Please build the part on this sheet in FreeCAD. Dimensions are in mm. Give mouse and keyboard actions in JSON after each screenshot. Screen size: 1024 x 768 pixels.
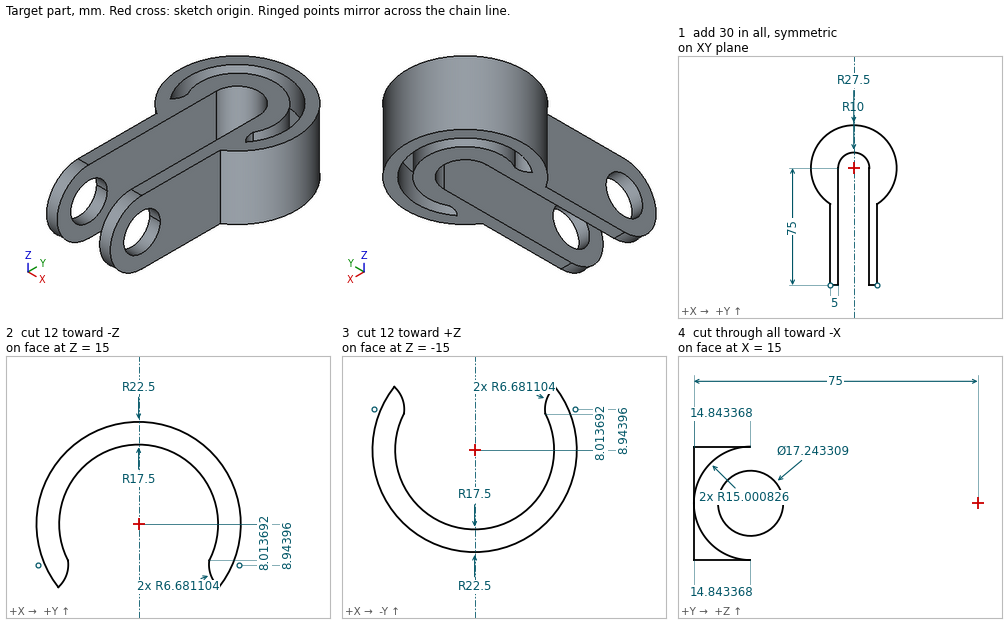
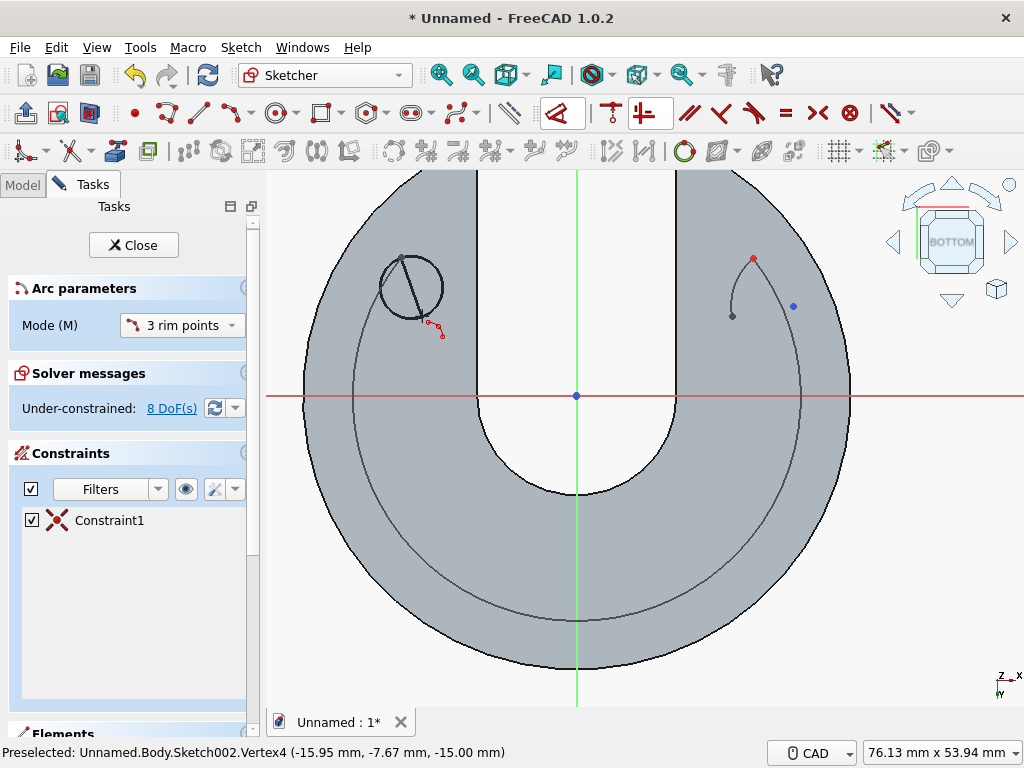
{"action": "scroll", "coordinate": [419, 284], "scroll_direction": "up", "scroll_amount": 4}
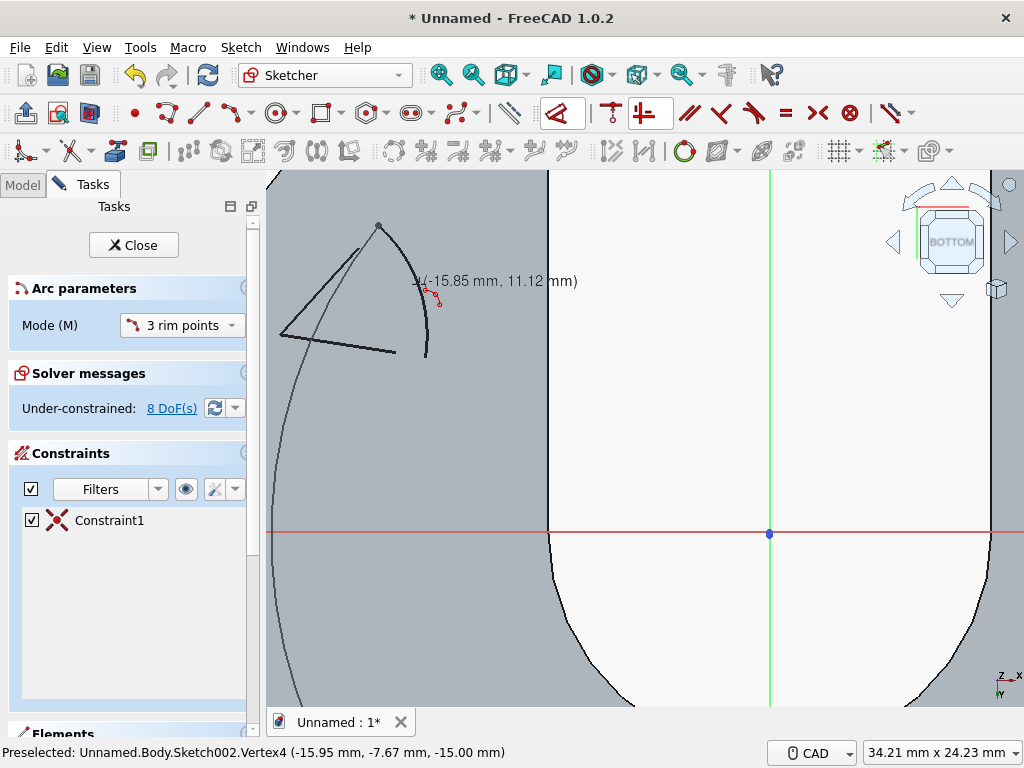
{"action": "left_click", "coordinate": [418, 284]}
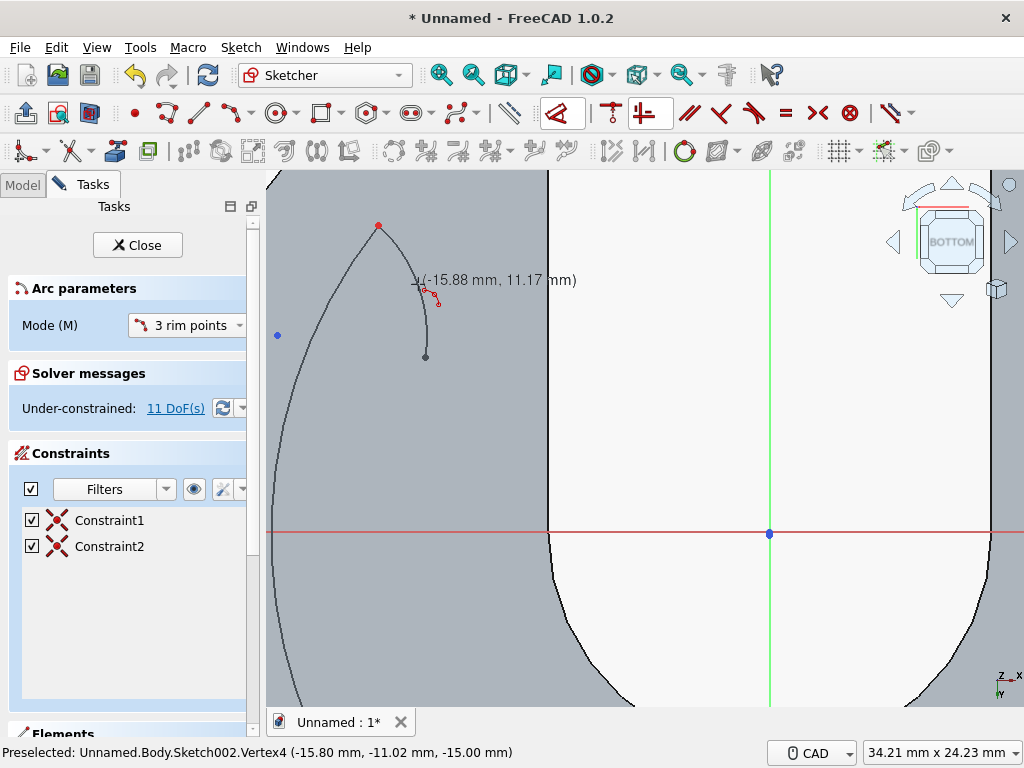
{"action": "left_click", "coordinate": [425, 357]}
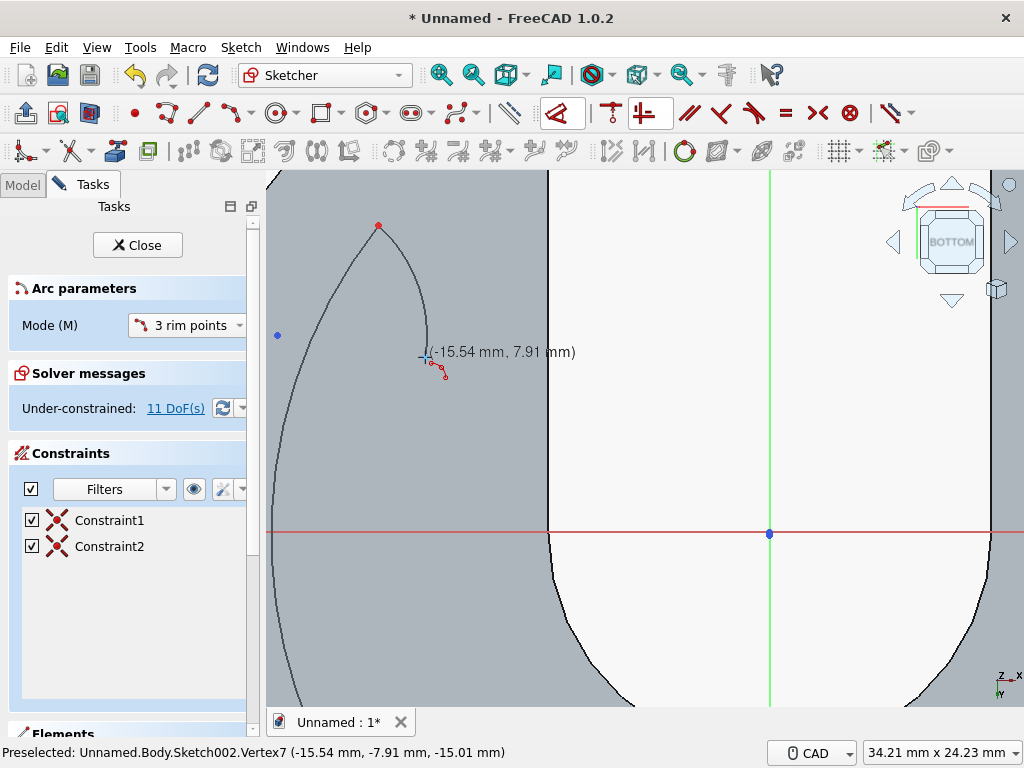
{"action": "scroll", "coordinate": [419, 284], "scroll_direction": "down", "scroll_amount": 4}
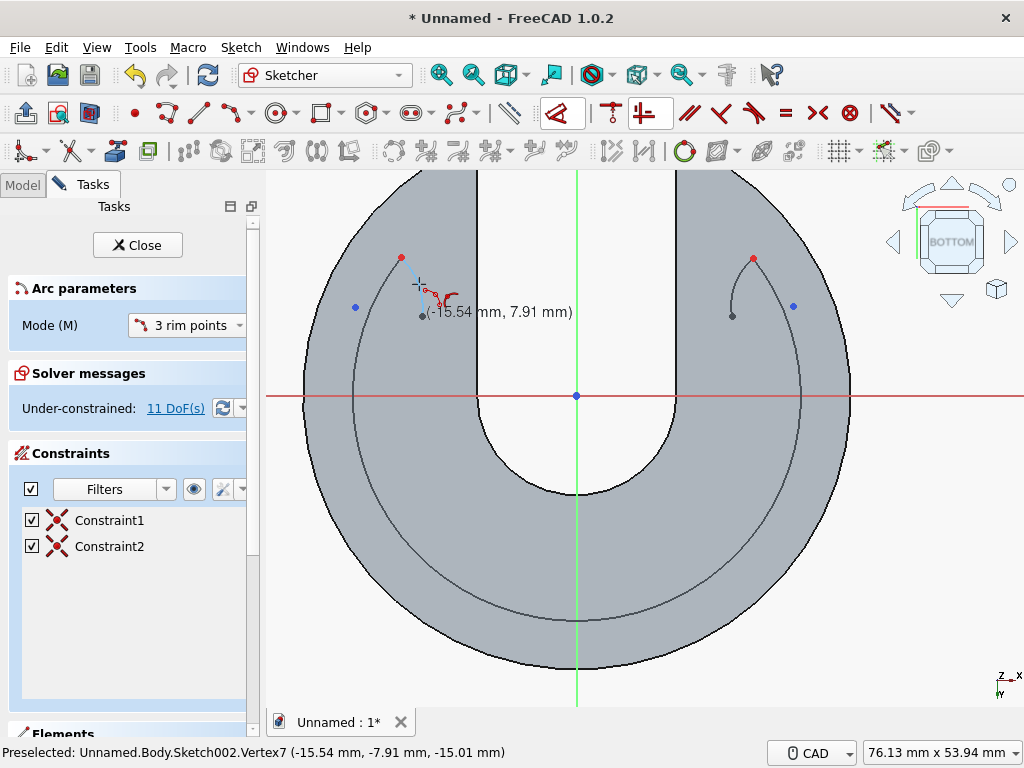
{"action": "left_click", "coordinate": [732, 317]}
{"action": "left_click", "coordinate": [507, 556]}
{"action": "key", "text": "Escape"}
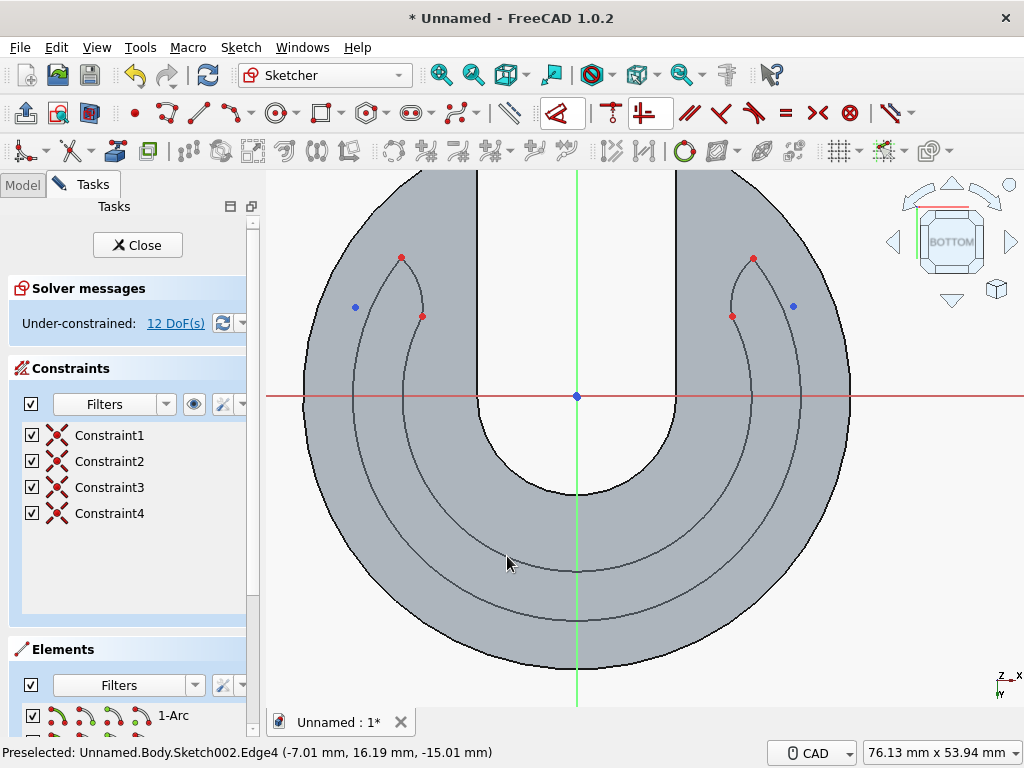
{"action": "left_click", "coordinate": [402, 537]}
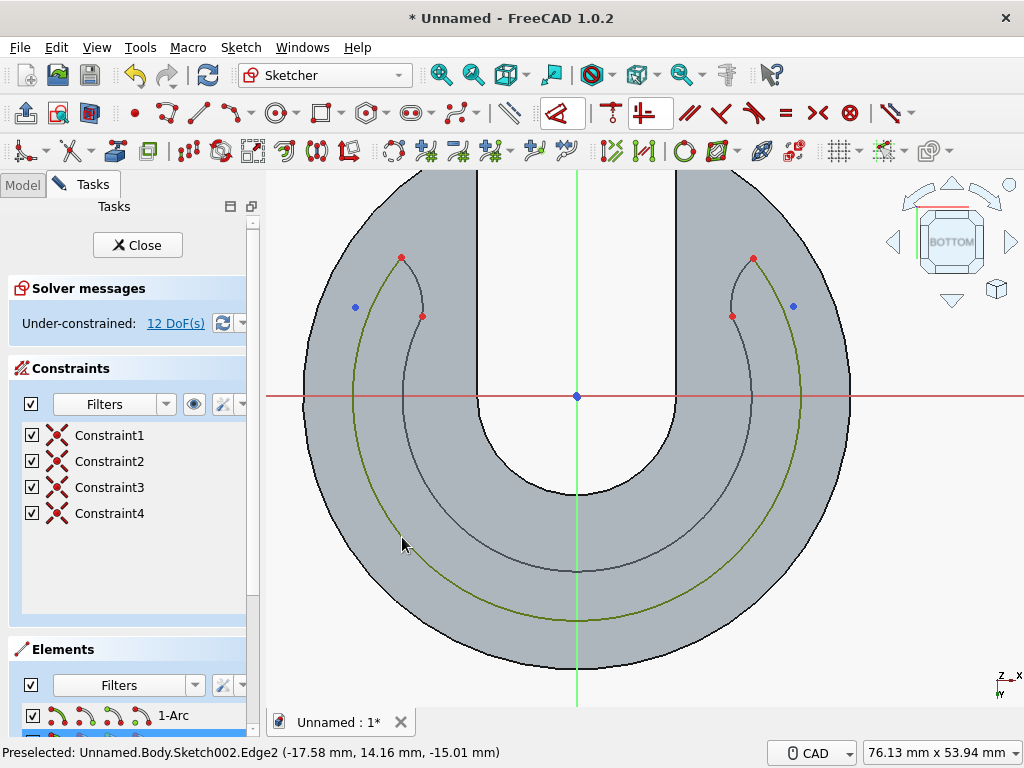
{"action": "left_click", "coordinate": [450, 516]}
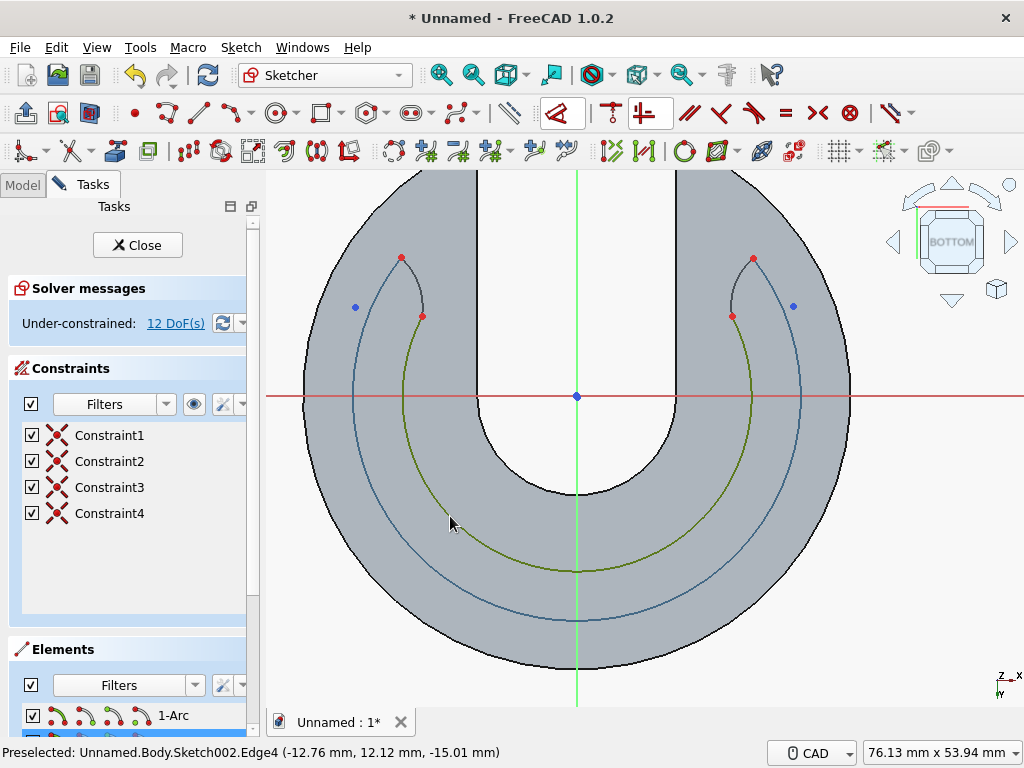
{"action": "key", "text": "c"}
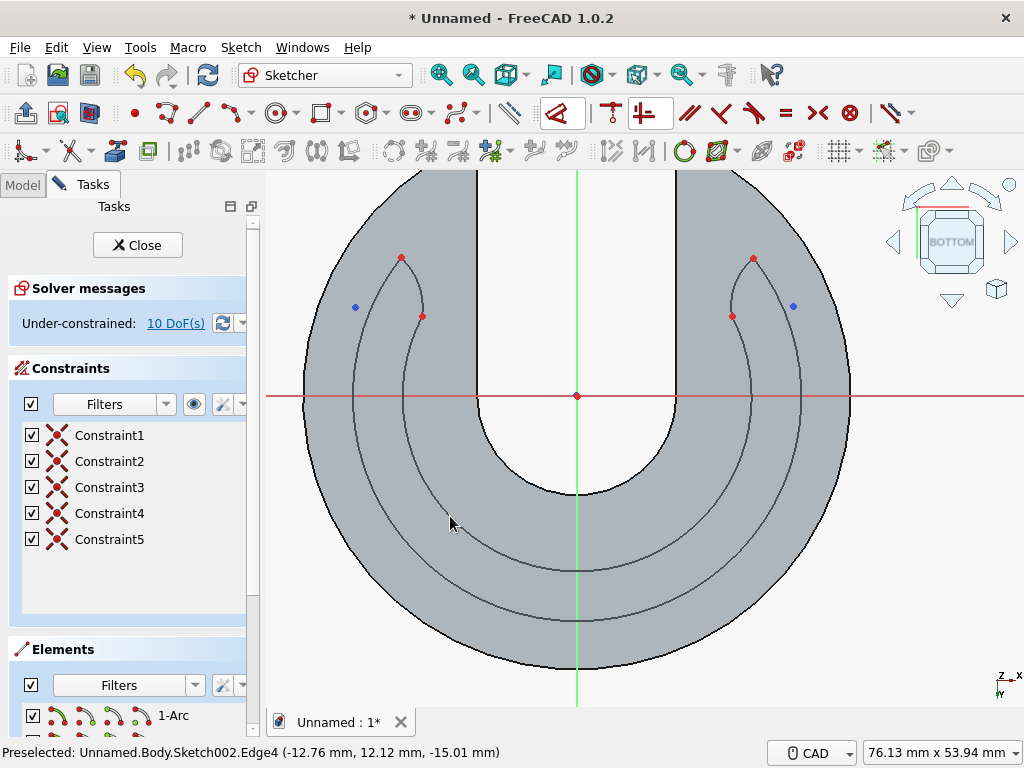
{"action": "left_click_drag", "start_coordinate": [567, 386], "coordinate": [587, 407]}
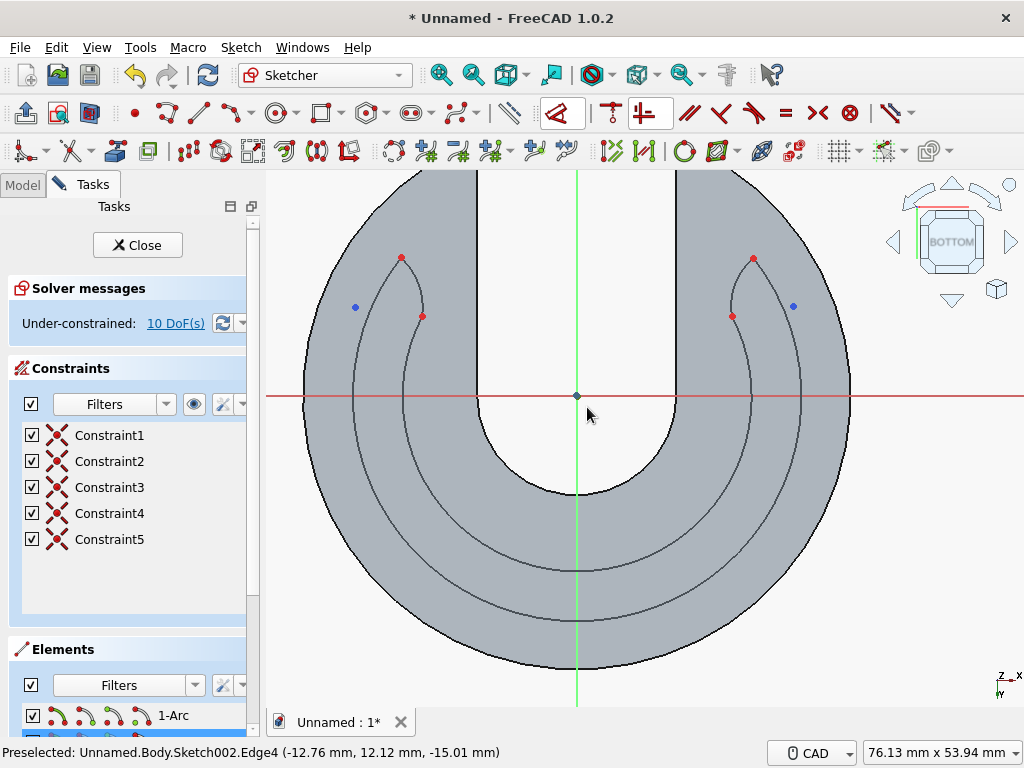
{"action": "left_click", "coordinate": [612, 114]}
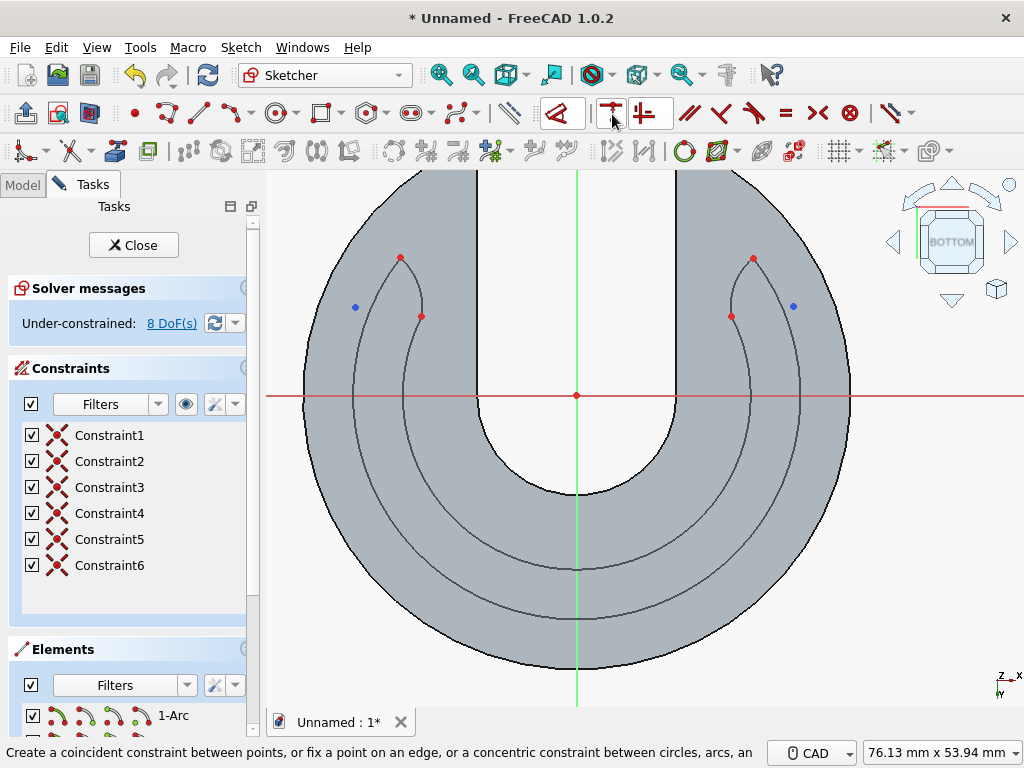
{"action": "left_click", "coordinate": [740, 273]}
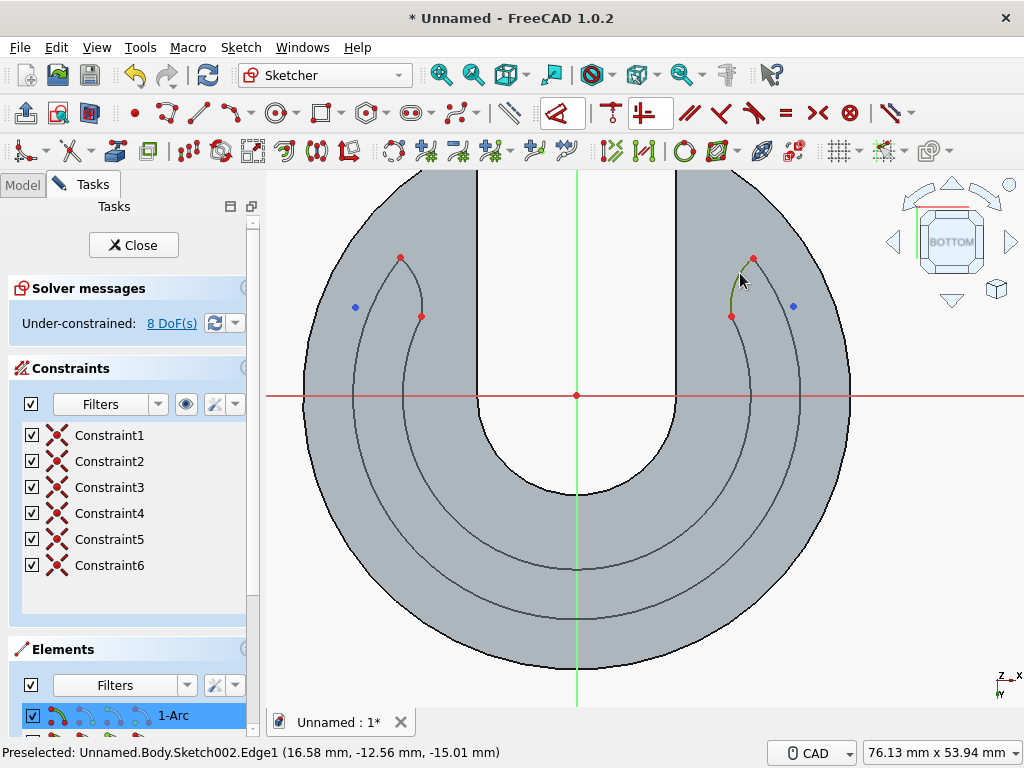
{"action": "left_click", "coordinate": [422, 297]}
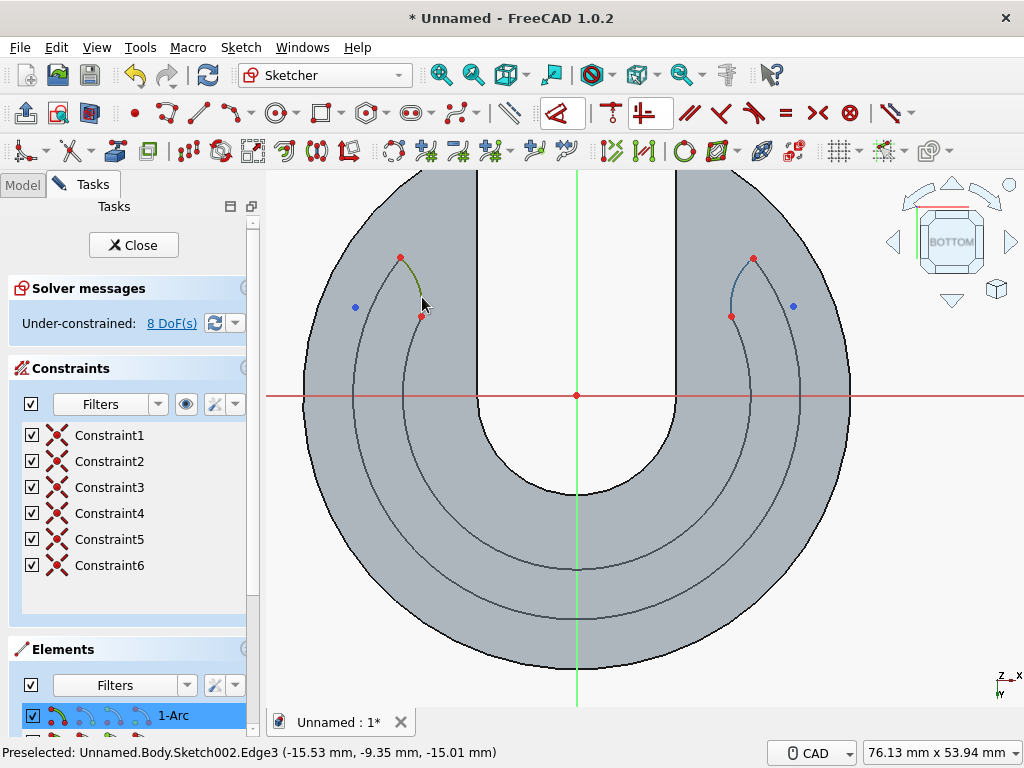
{"action": "key", "text": "e"}